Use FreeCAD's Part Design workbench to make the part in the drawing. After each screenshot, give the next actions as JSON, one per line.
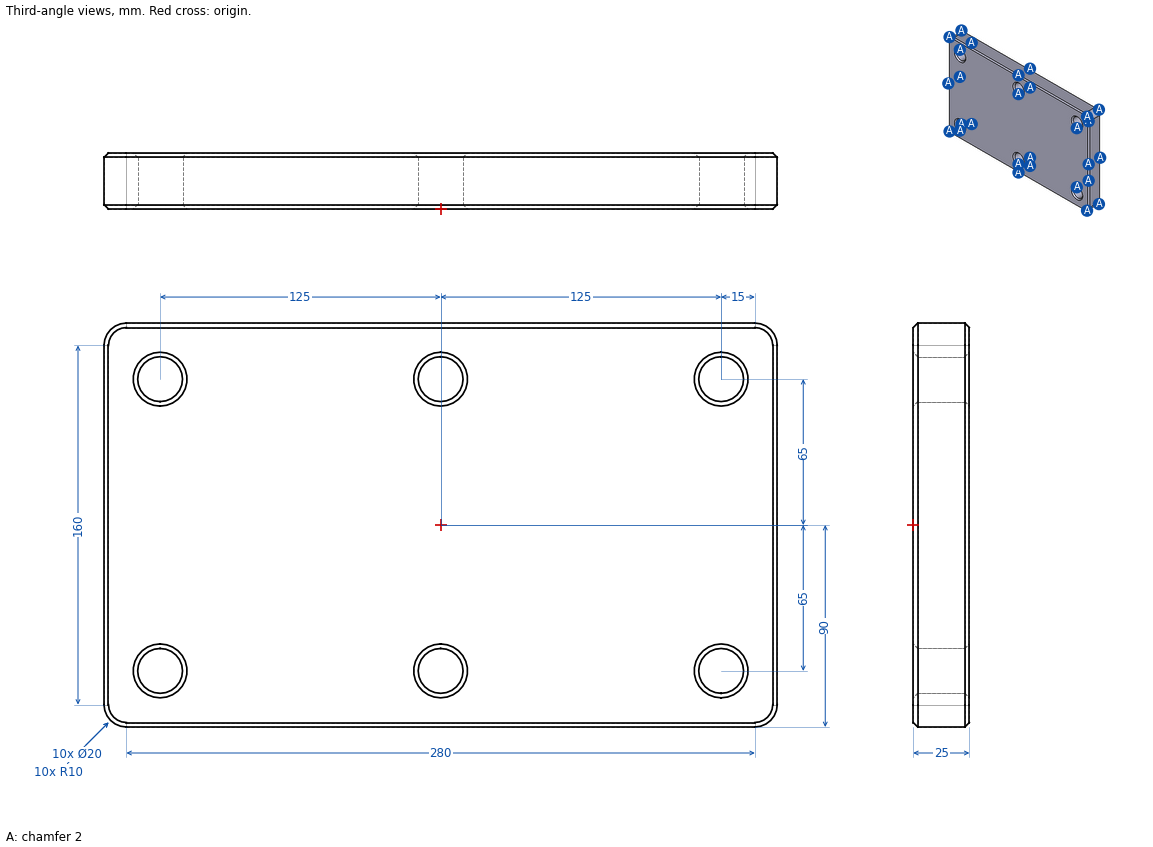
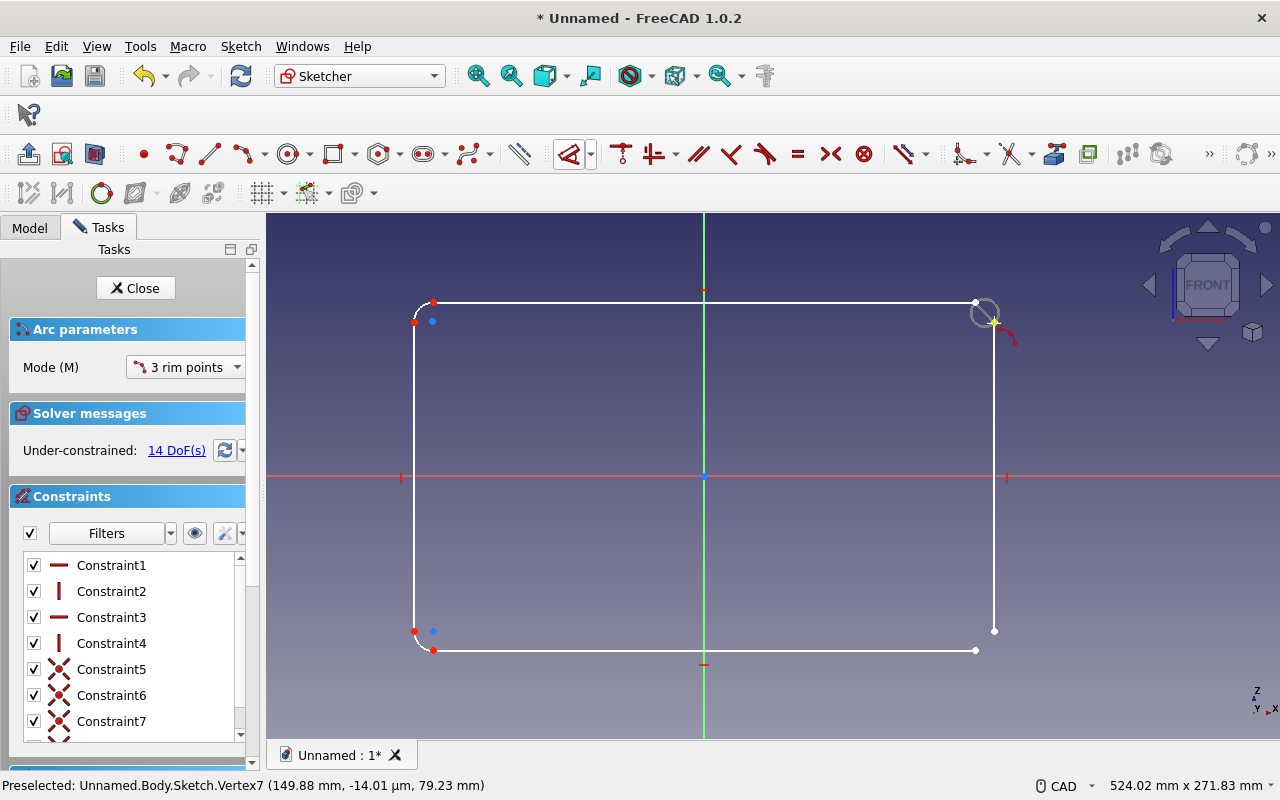
{"action": "scroll", "coordinate": [989, 308], "scroll_direction": "up", "scroll_amount": 6}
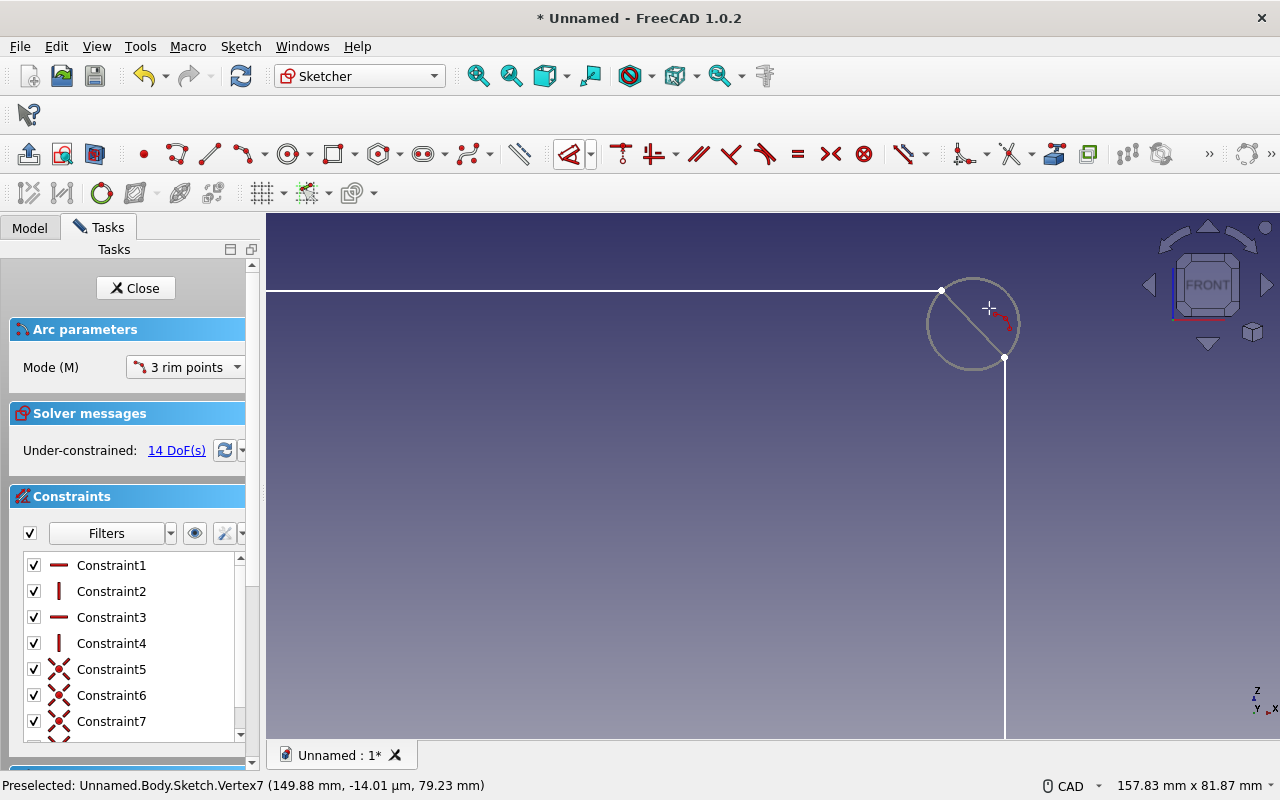
{"action": "left_click", "coordinate": [987, 307]}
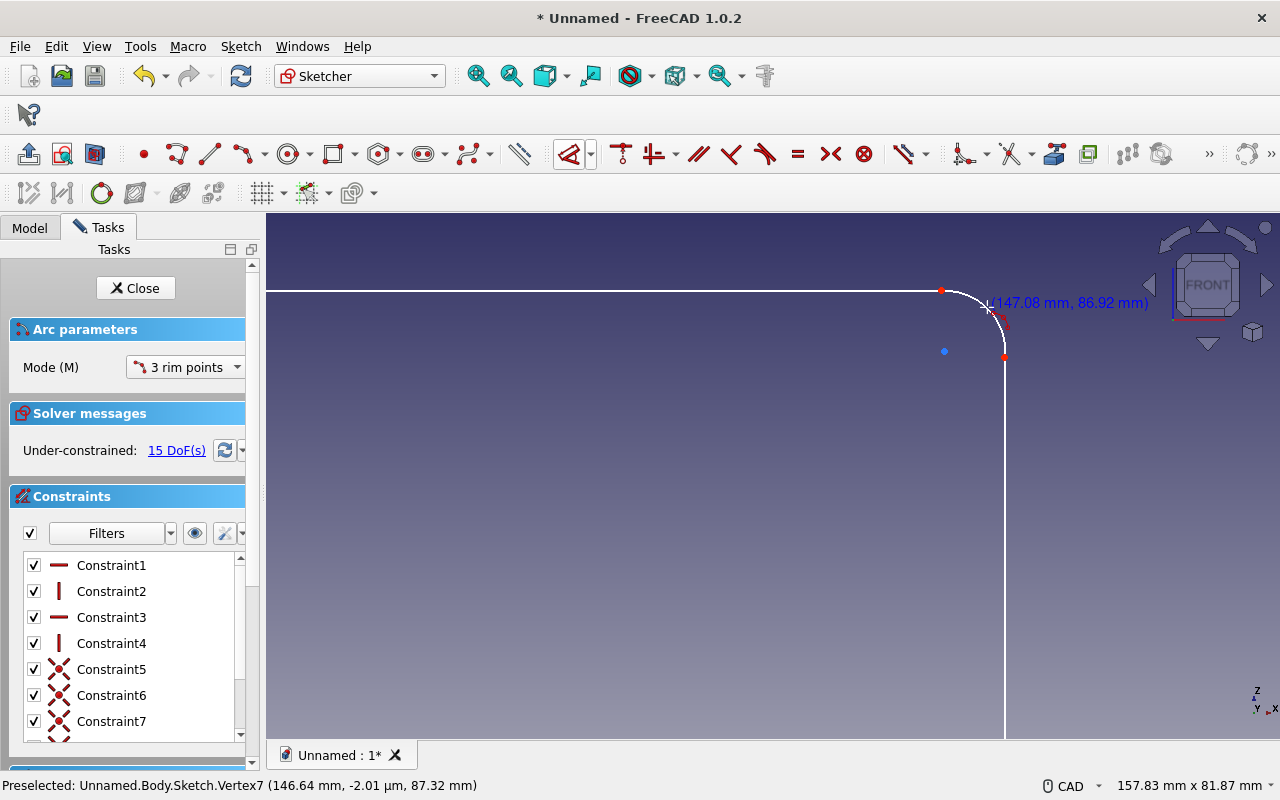
{"action": "scroll", "coordinate": [990, 308], "scroll_direction": "down", "scroll_amount": 6}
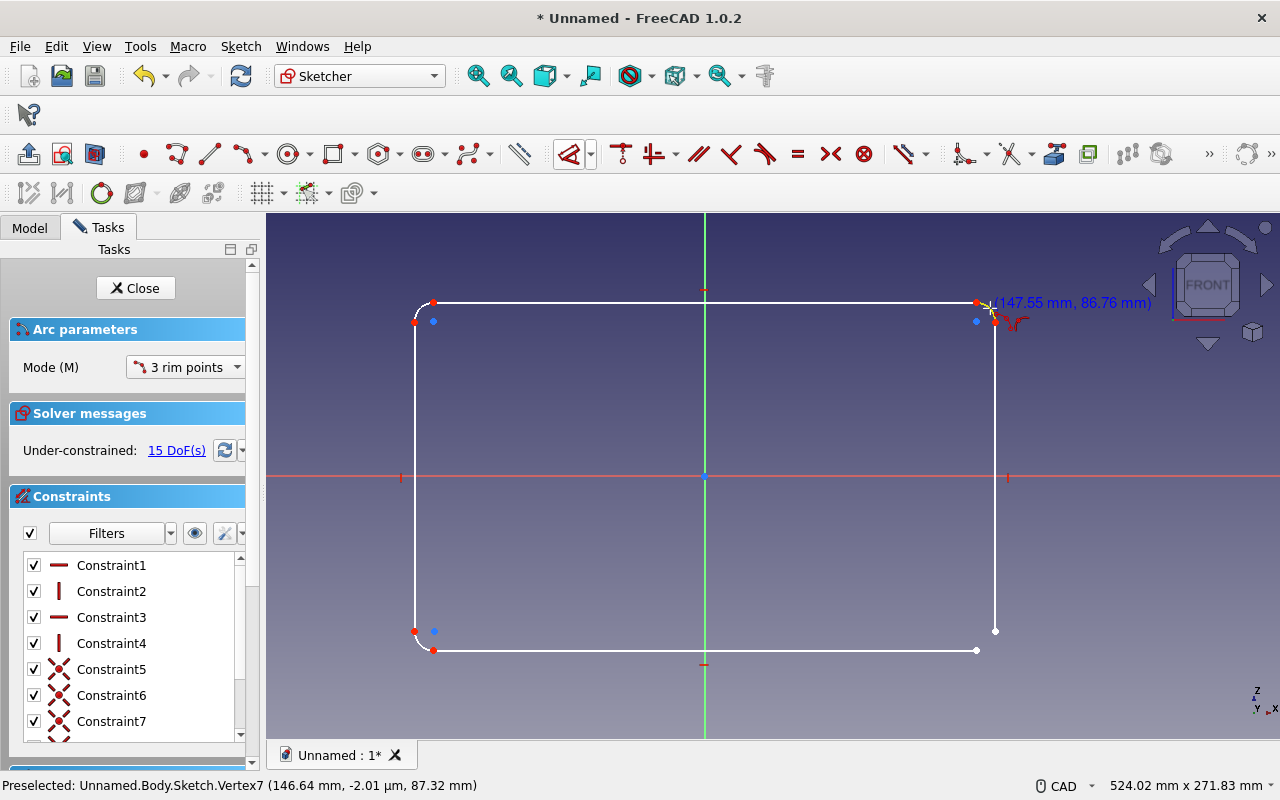
{"action": "left_click", "coordinate": [995, 632]}
{"action": "left_click", "coordinate": [976, 651]}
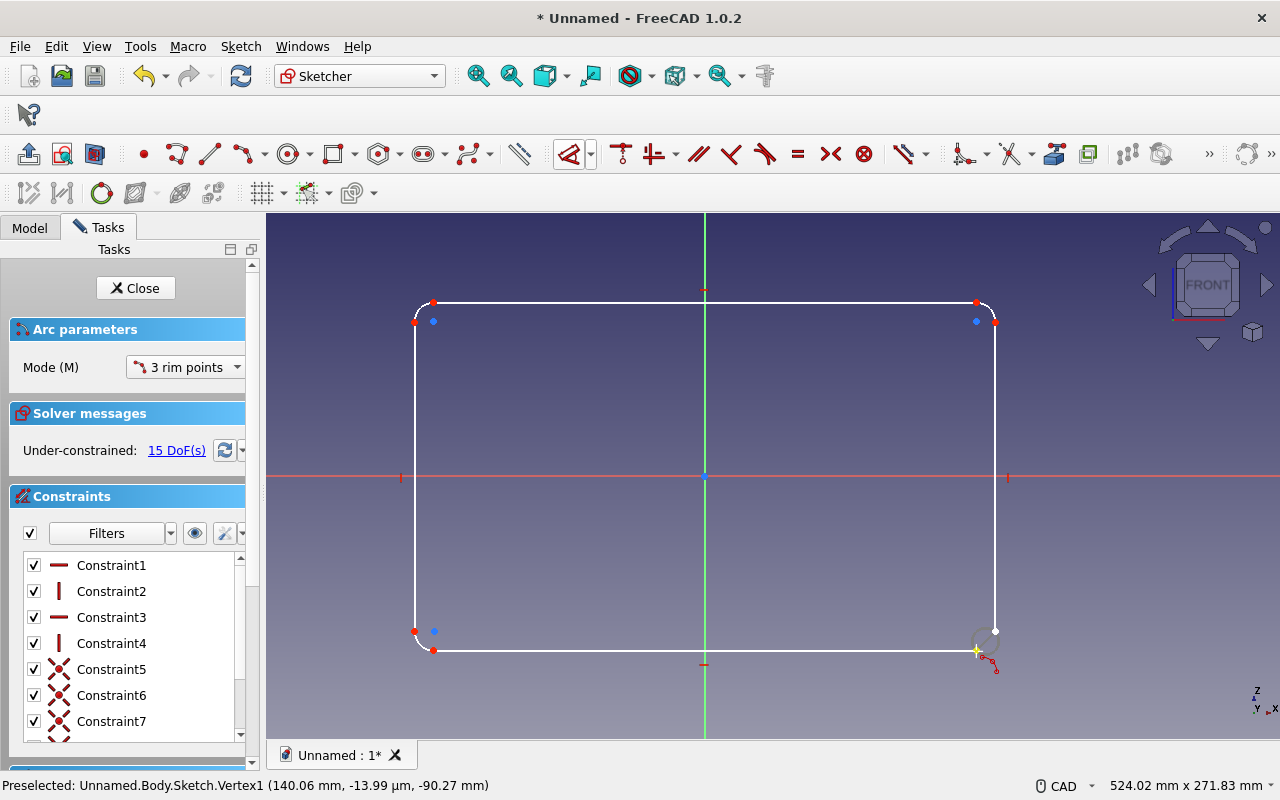
{"action": "scroll", "coordinate": [990, 645], "scroll_direction": "up", "scroll_amount": 6}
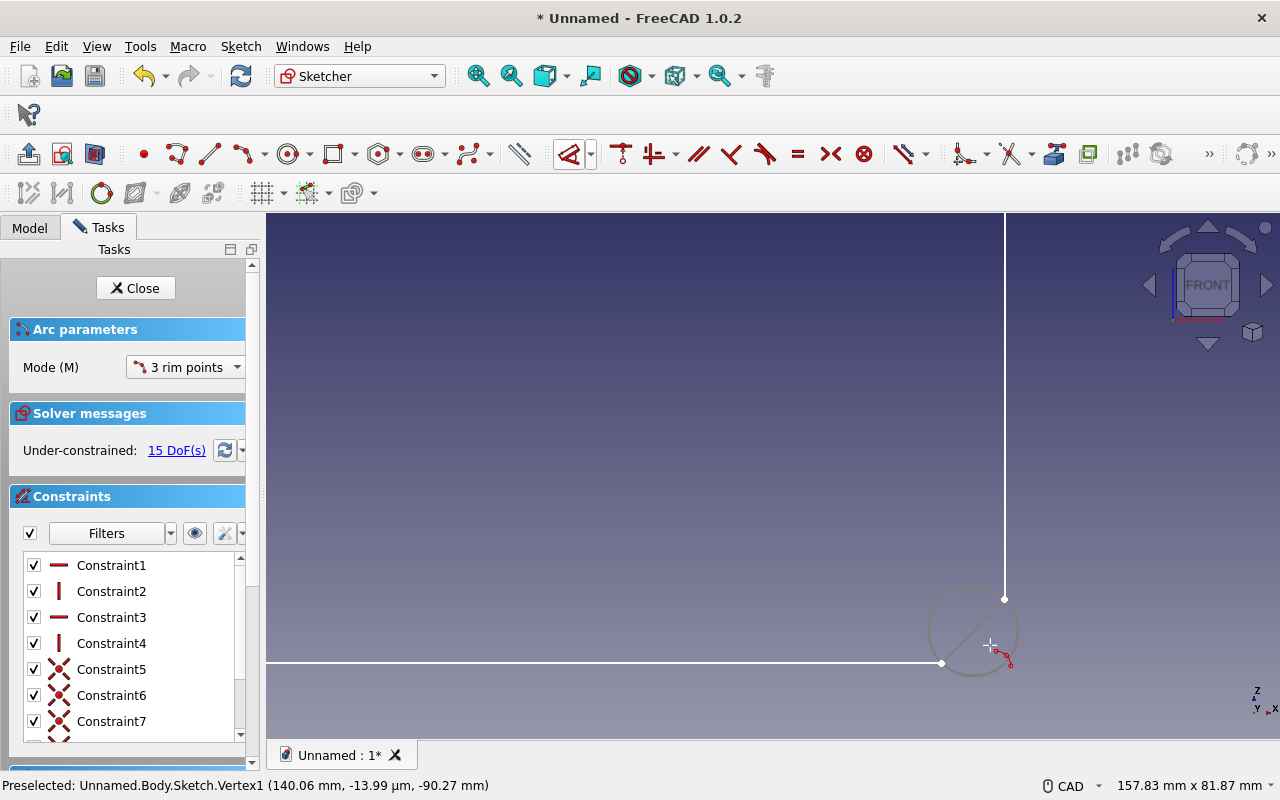
{"action": "left_click", "coordinate": [987, 642]}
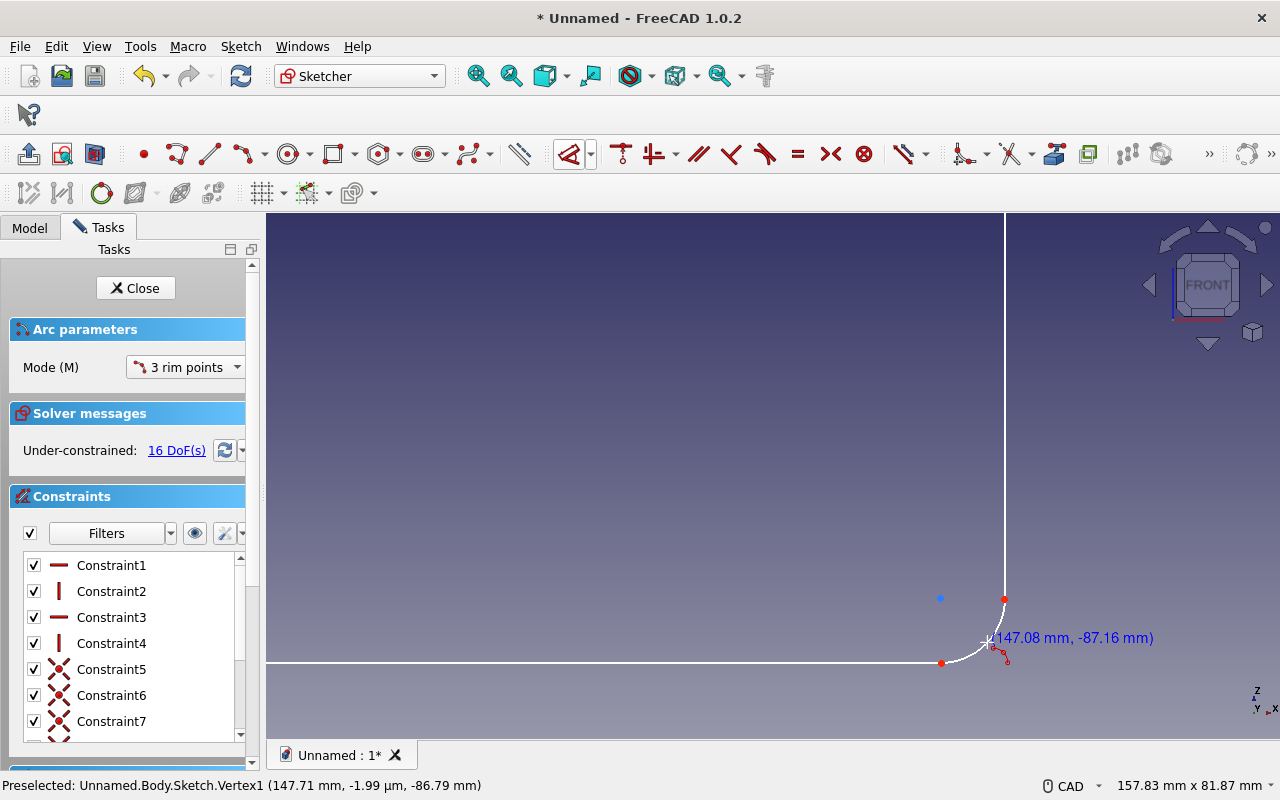
{"action": "left_click", "coordinate": [288, 154]}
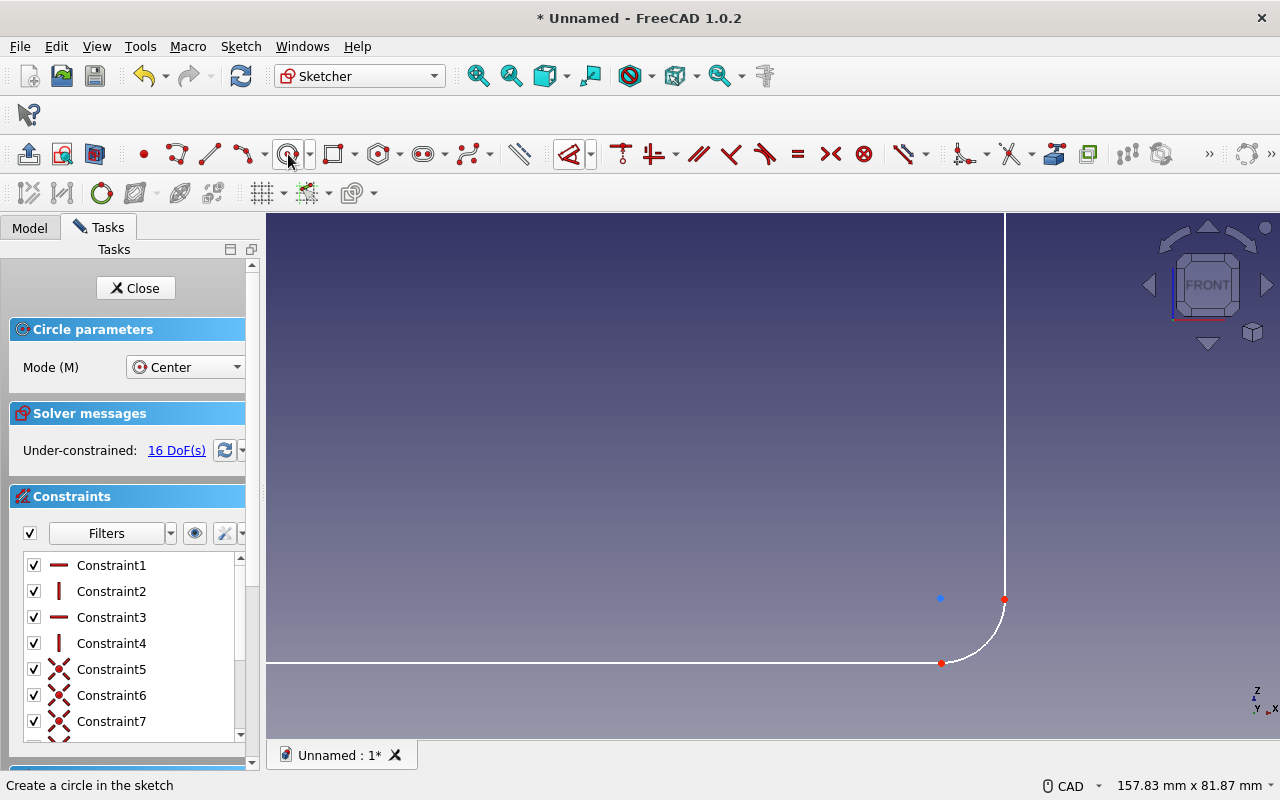
{"action": "scroll", "coordinate": [990, 645], "scroll_direction": "down", "scroll_amount": 6}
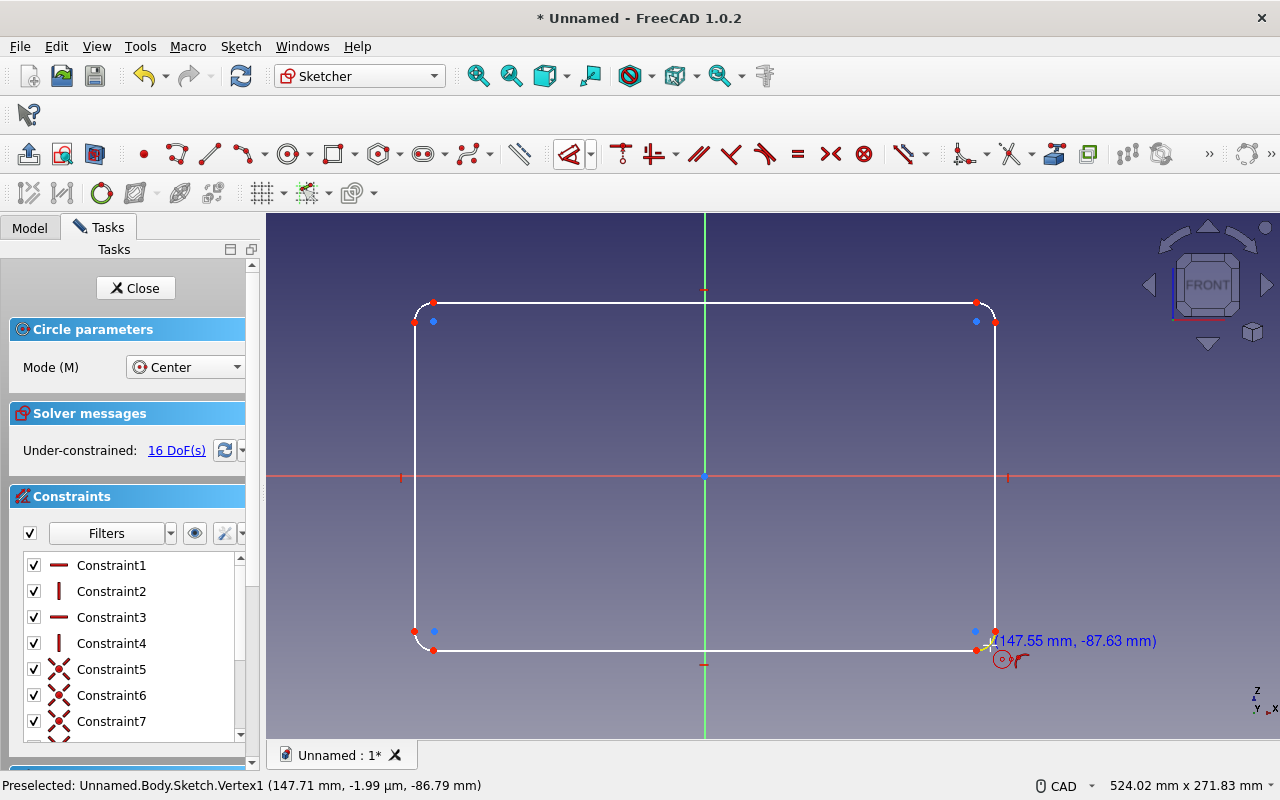
{"action": "left_click", "coordinate": [947, 351]}
{"action": "left_click", "coordinate": [961, 337]}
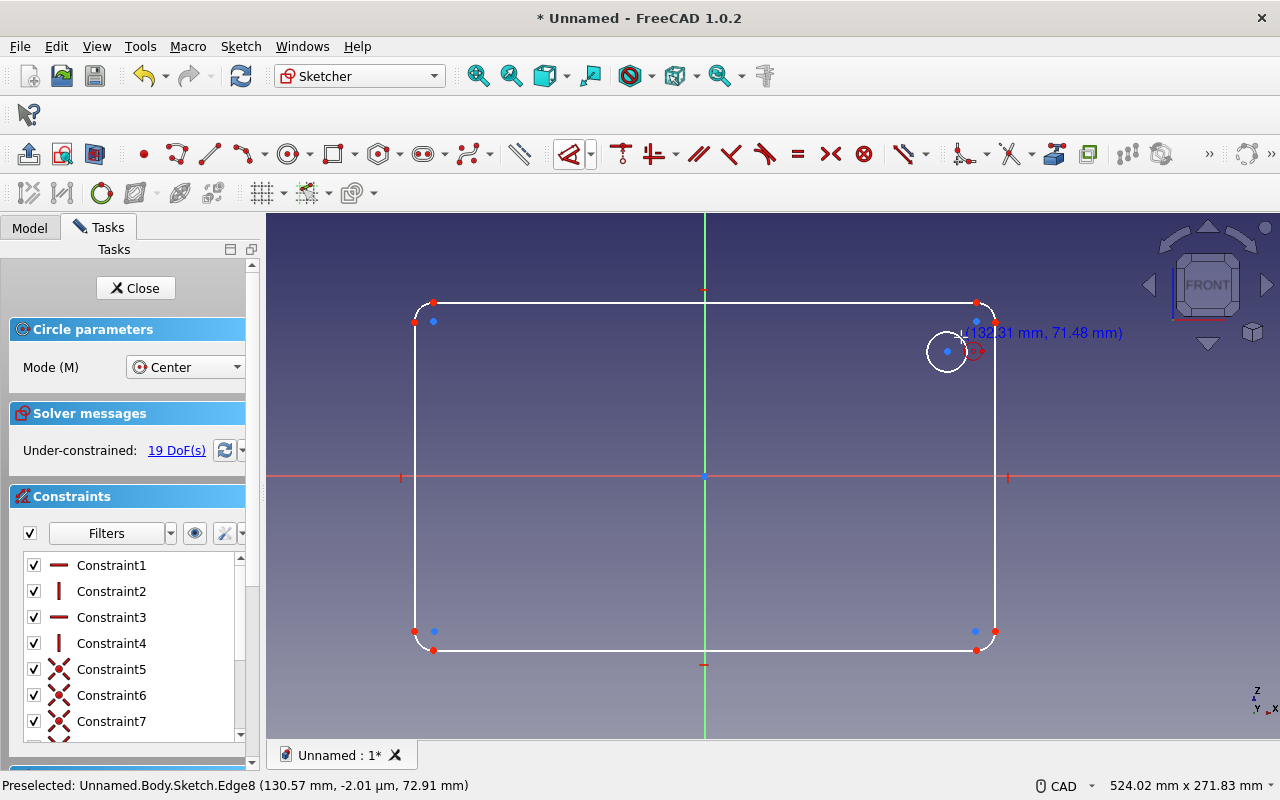
{"action": "left_click", "coordinate": [705, 351]}
{"action": "left_click", "coordinate": [723, 344]}